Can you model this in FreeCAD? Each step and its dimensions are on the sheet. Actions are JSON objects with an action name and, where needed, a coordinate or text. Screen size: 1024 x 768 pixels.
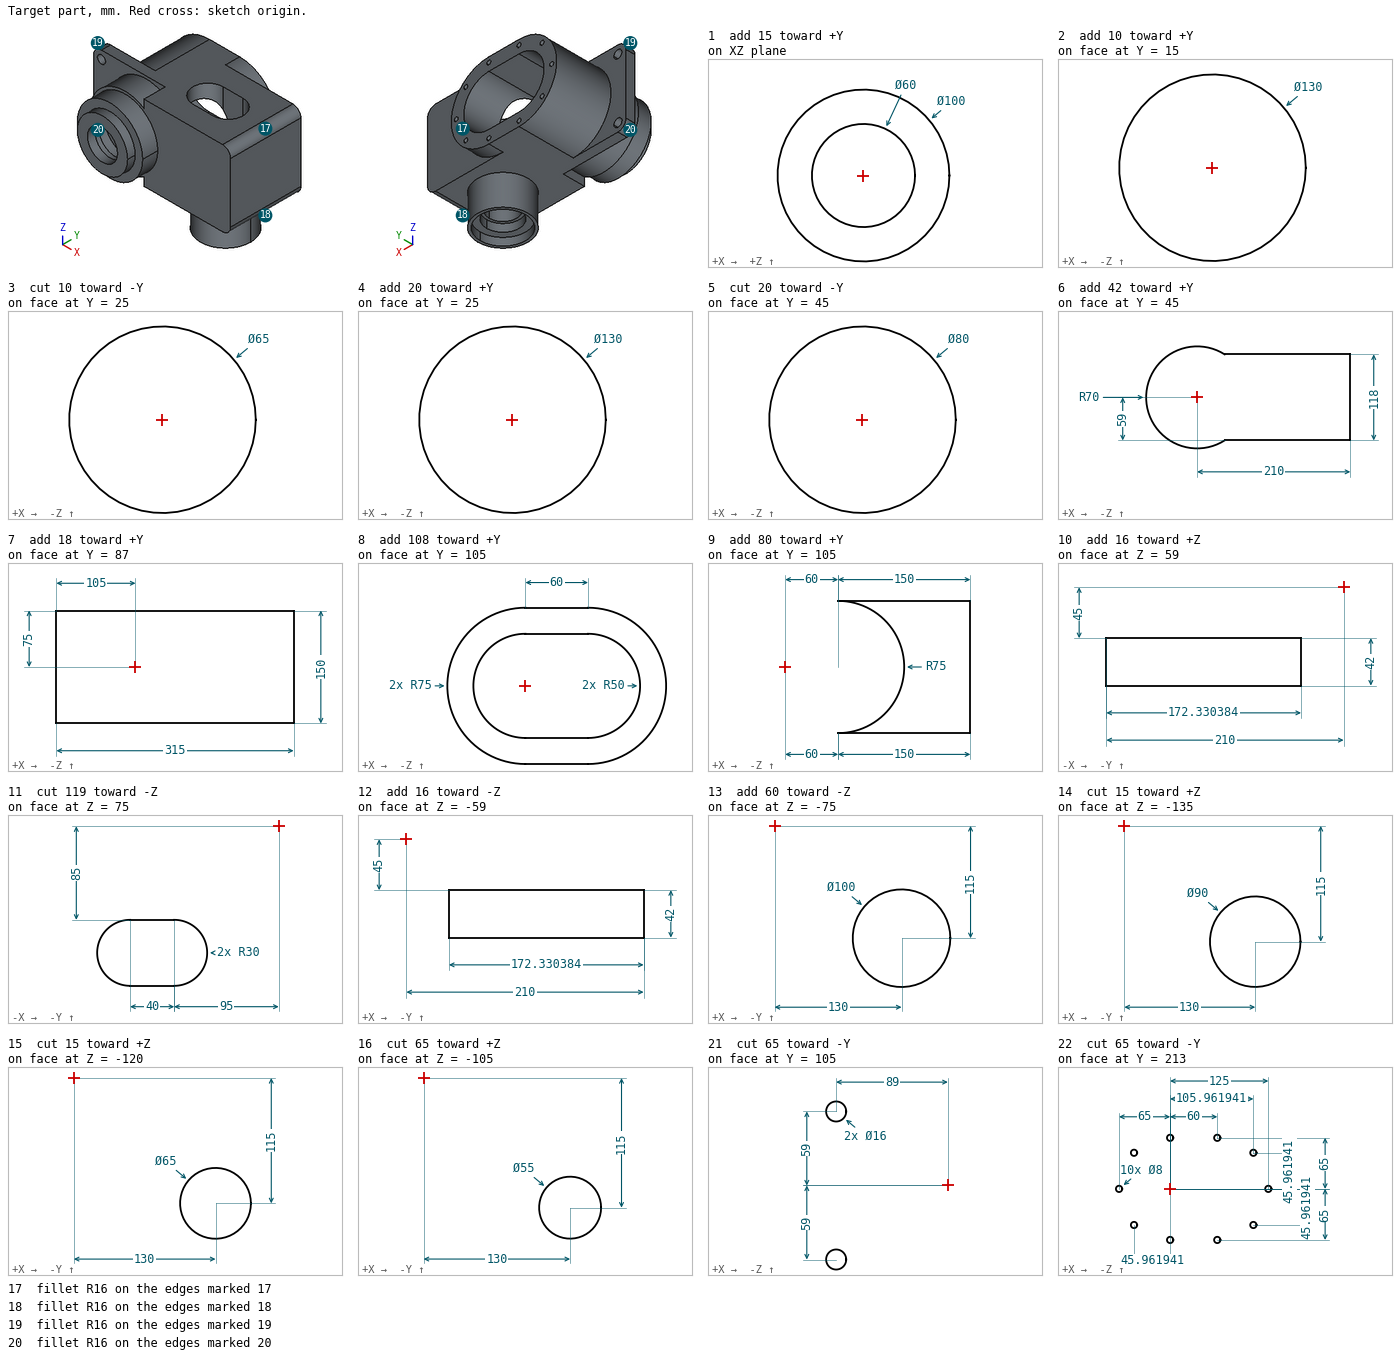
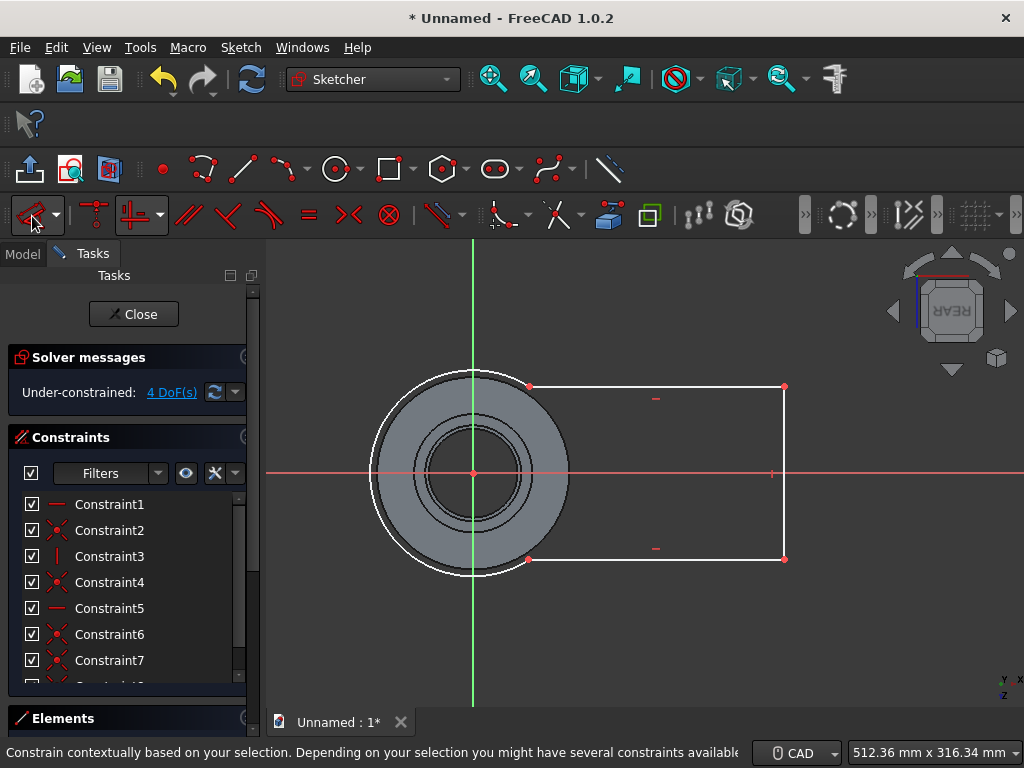
{"action": "left_click", "coordinate": [406, 395]}
{"action": "left_click", "coordinate": [385, 371]}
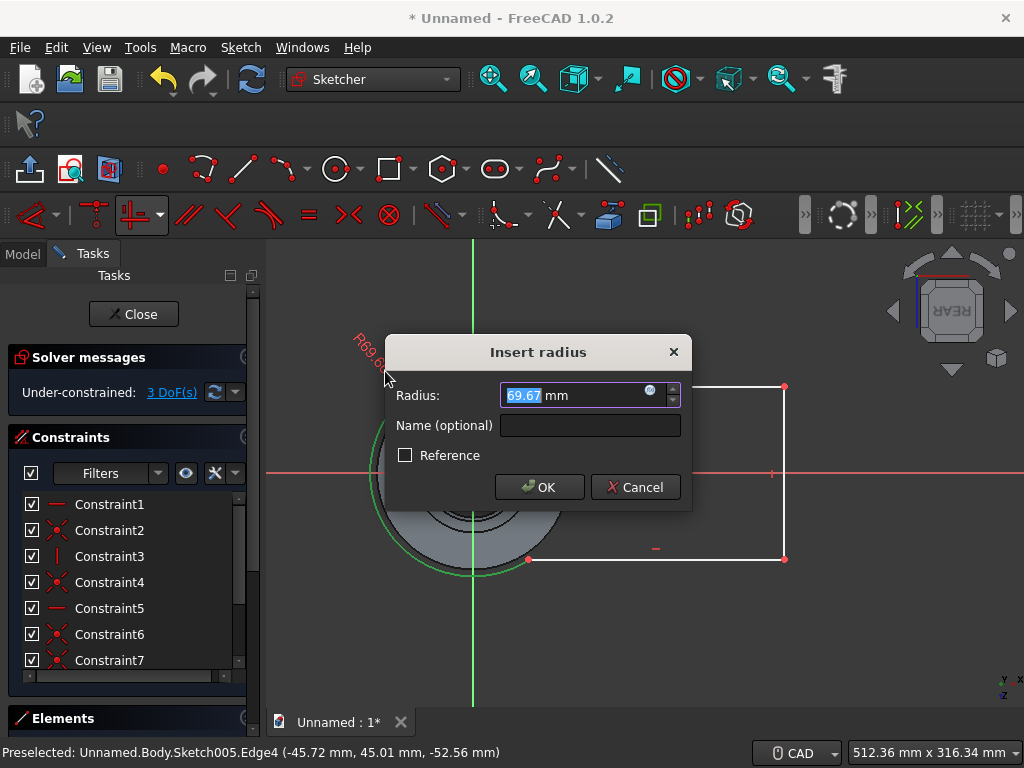
{"action": "type", "text": "70"}
{"action": "key", "text": "Return"}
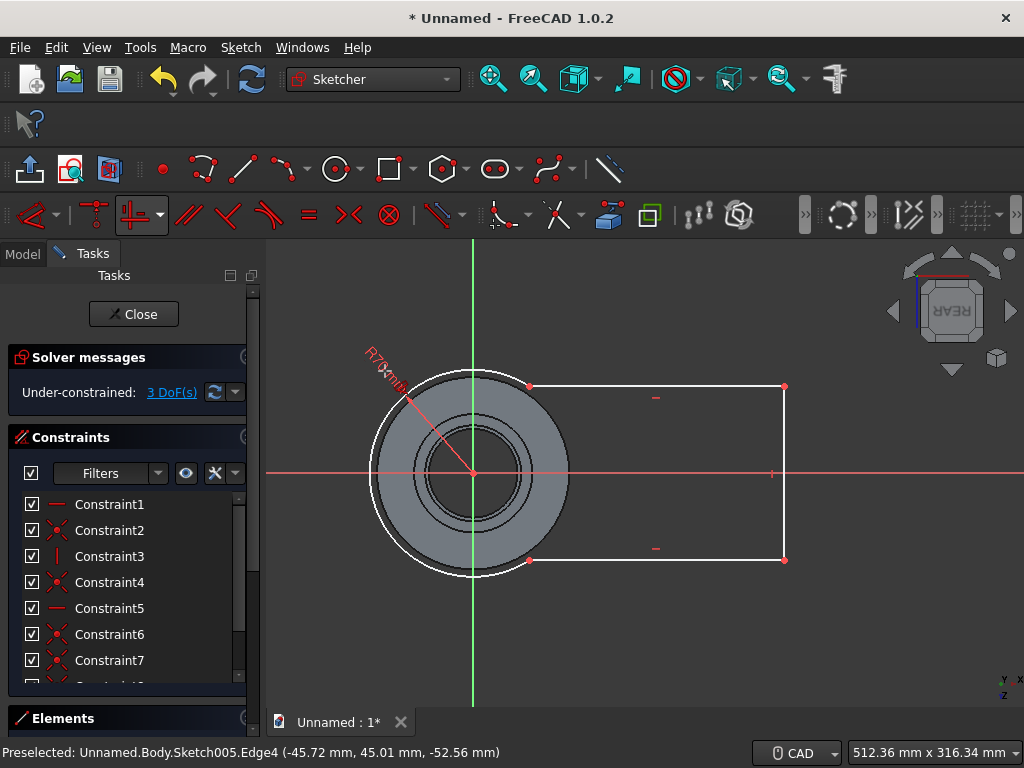
{"action": "left_click", "coordinate": [784, 508]}
{"action": "left_click", "coordinate": [818, 433]}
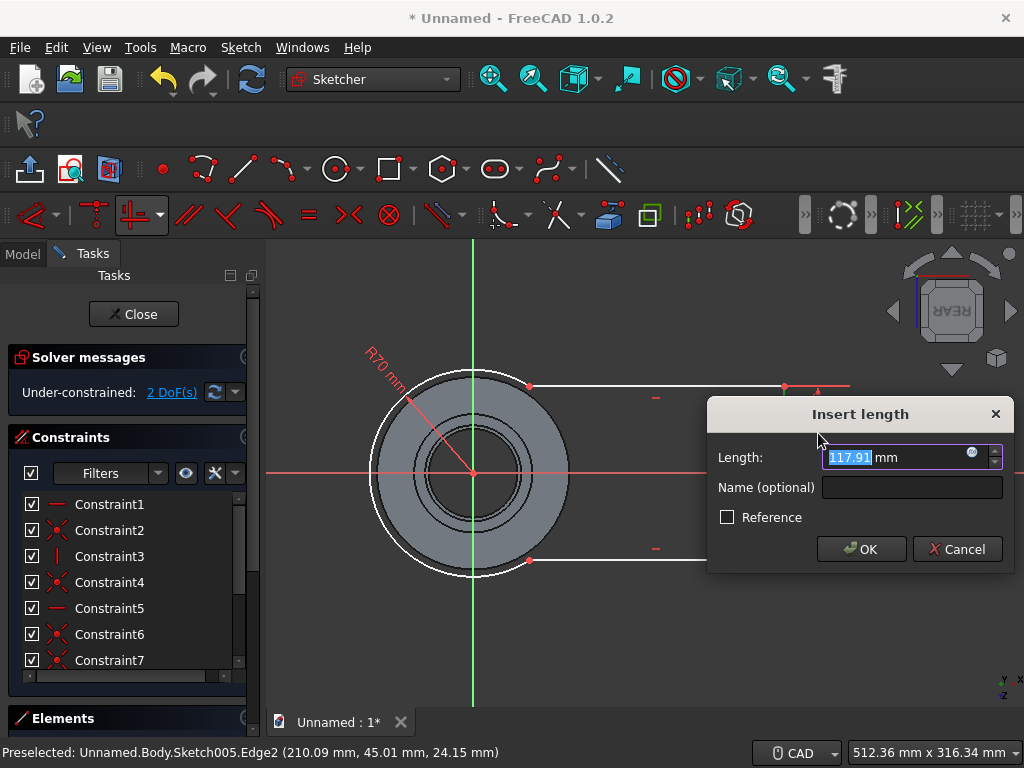
{"action": "type", "text": "118"}
{"action": "key", "text": "Return"}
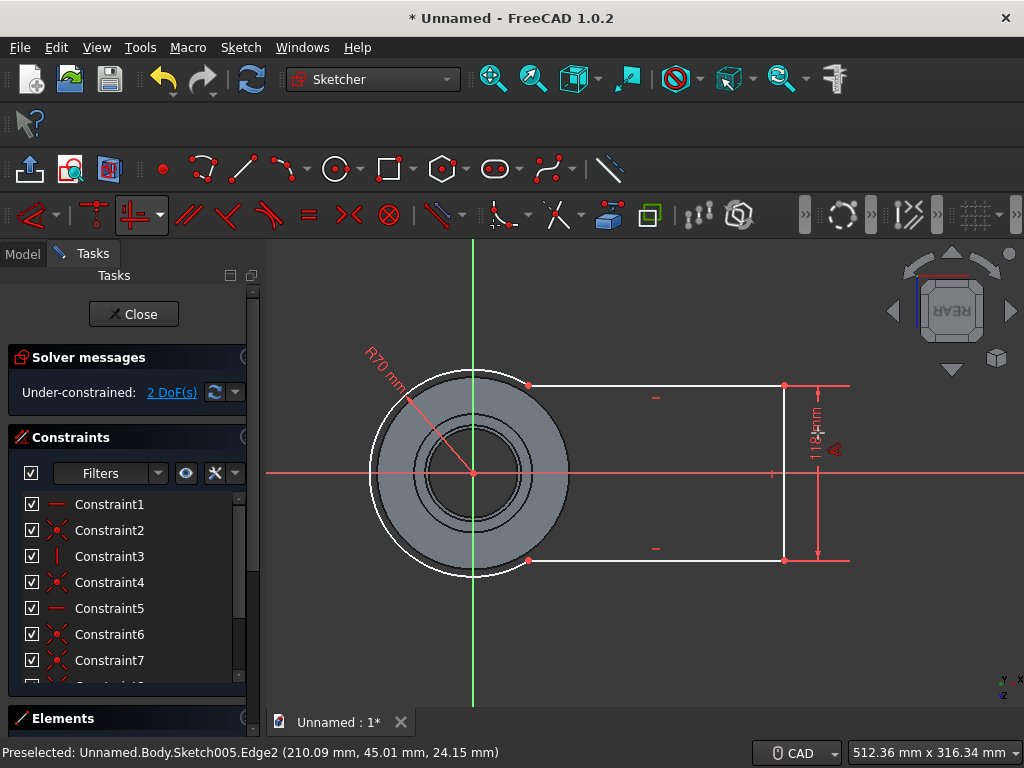
{"action": "left_click", "coordinate": [529, 561]}
{"action": "left_click", "coordinate": [439, 517]}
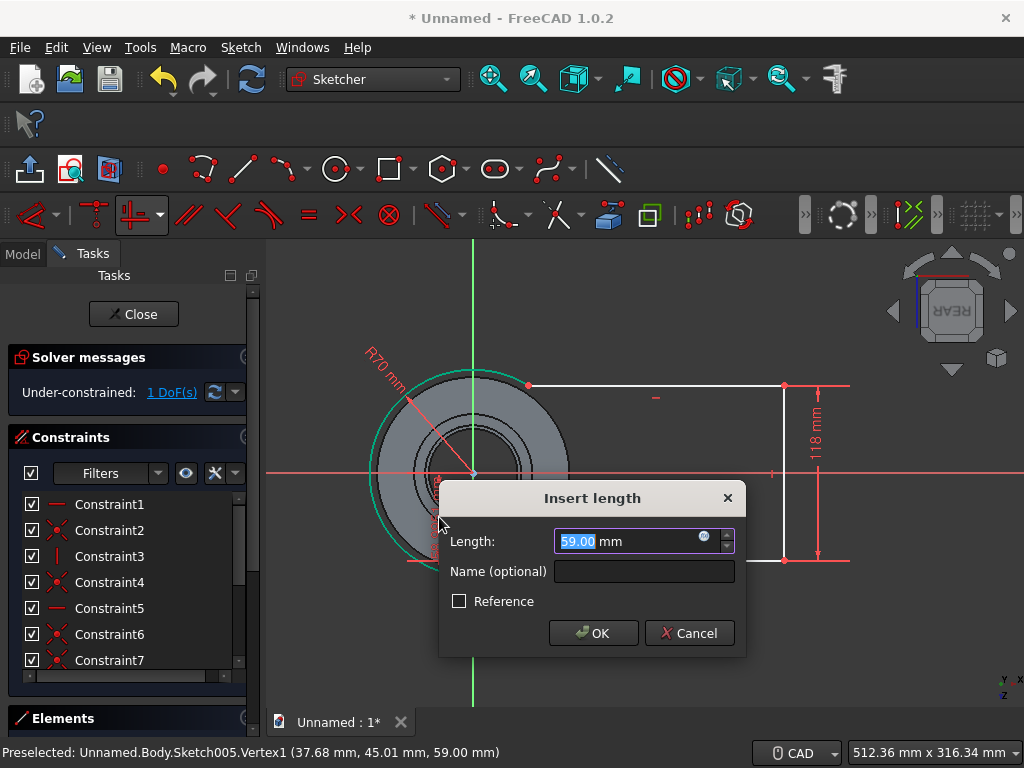
{"action": "type", "text": "59"}
{"action": "key", "text": "Return"}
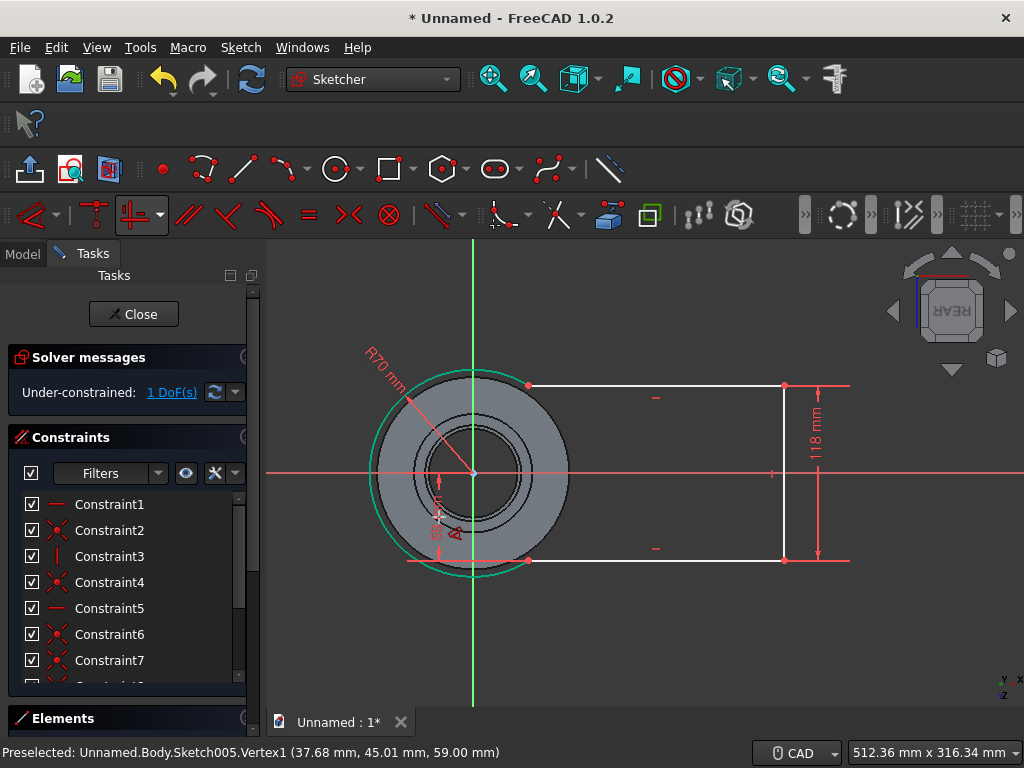
{"action": "left_click", "coordinate": [784, 561]}
{"action": "left_click", "coordinate": [629, 595]}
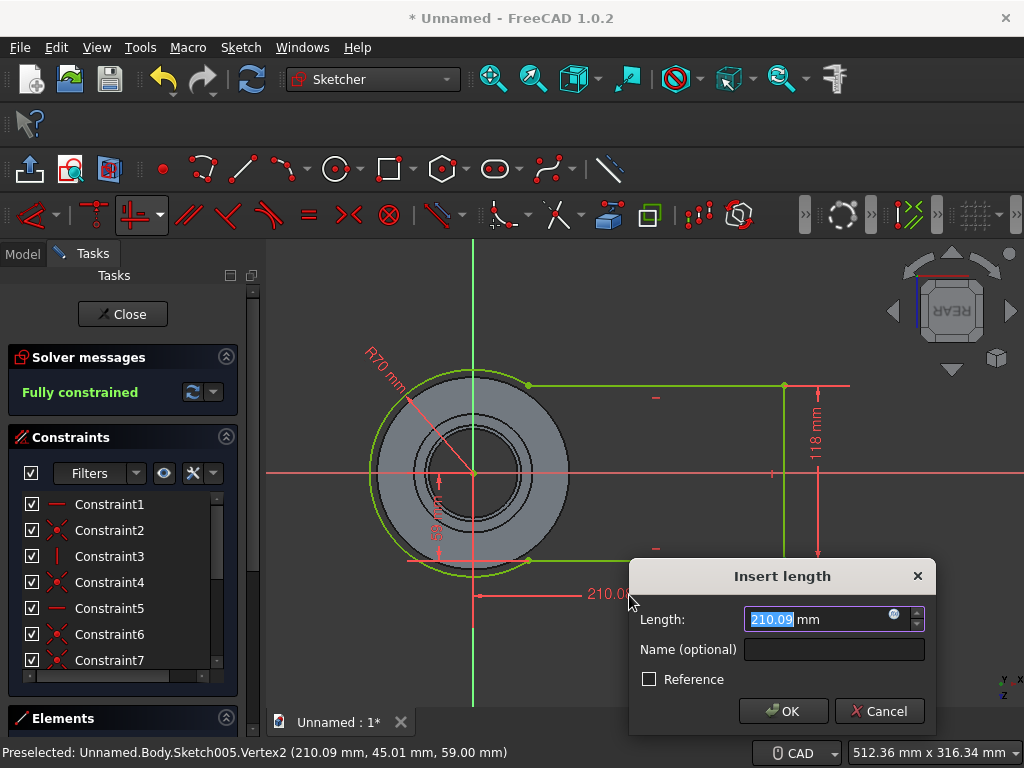
{"action": "type", "text": "210"}
{"action": "key", "text": "Return"}
{"action": "key", "text": "Escape"}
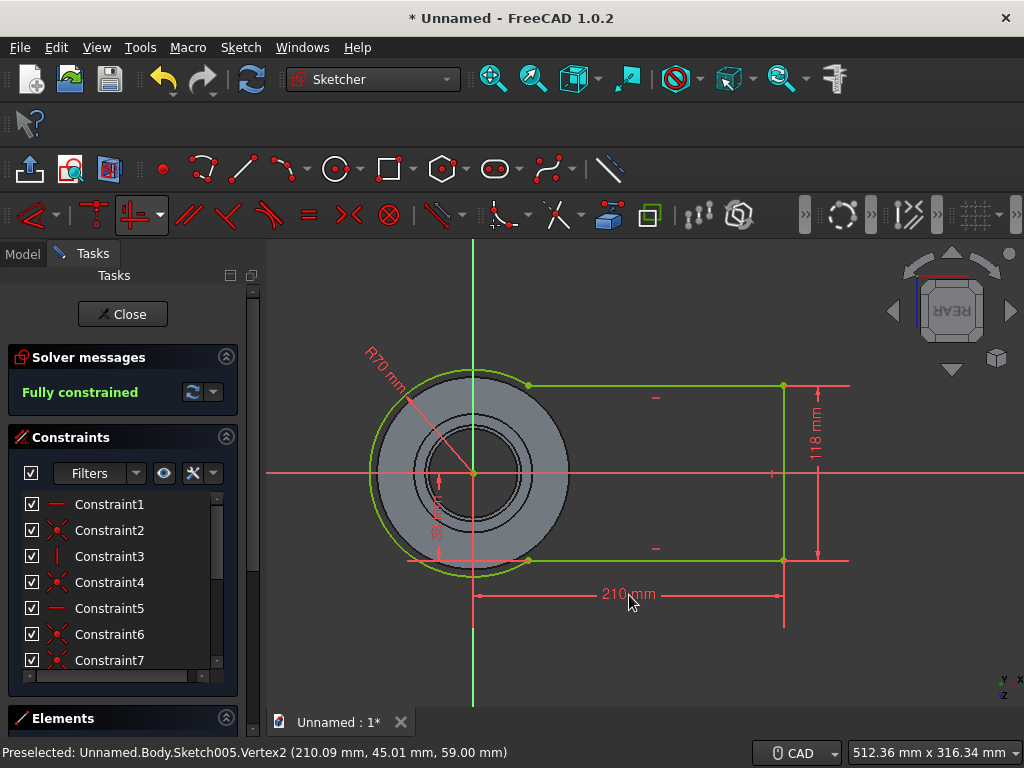
{"action": "left_click", "coordinate": [123, 314]}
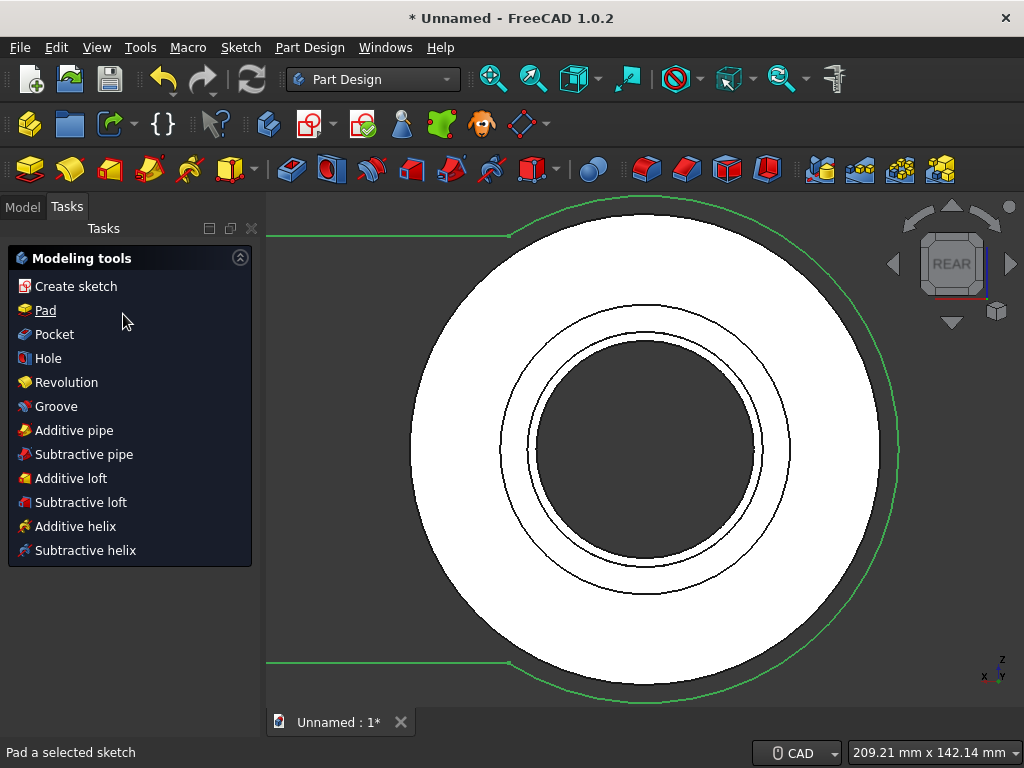
{"action": "left_click", "coordinate": [30, 170]}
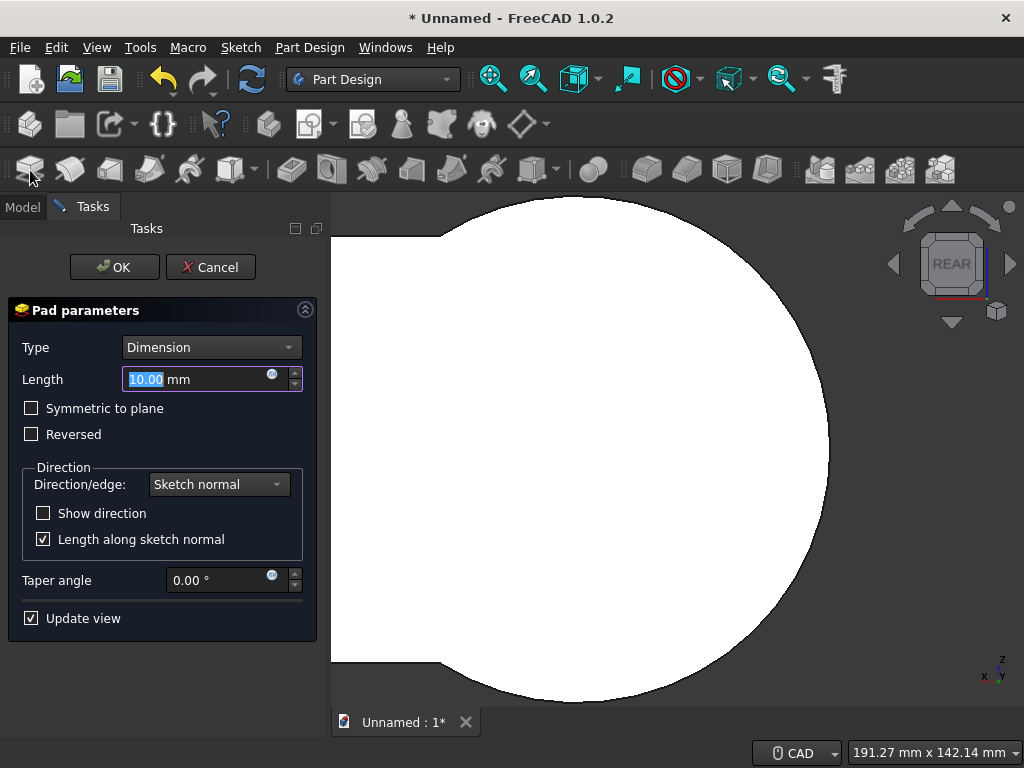
{"action": "type", "text": "42"}
{"action": "key", "text": "Tab"}